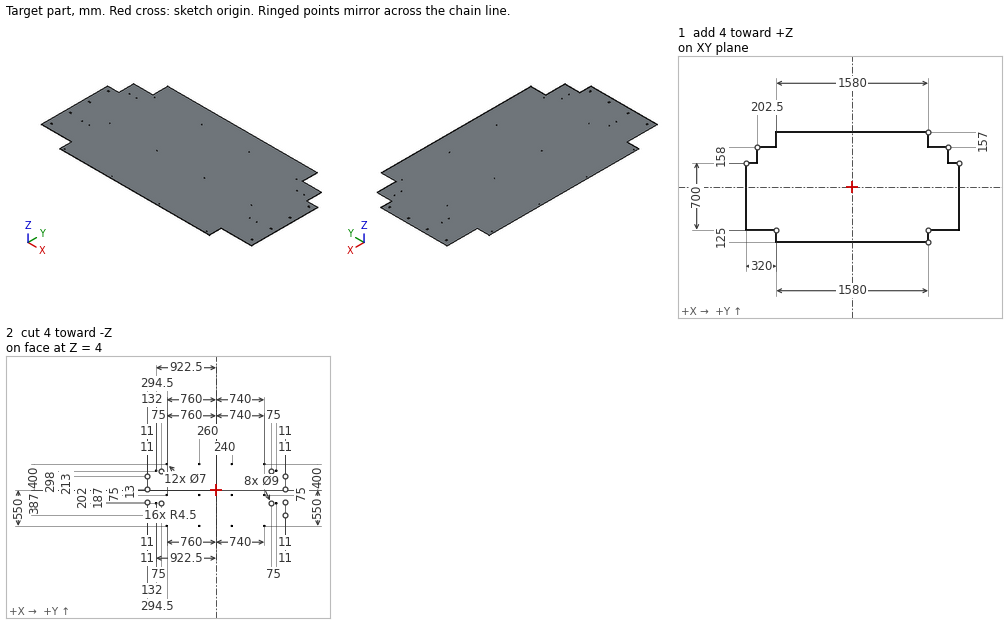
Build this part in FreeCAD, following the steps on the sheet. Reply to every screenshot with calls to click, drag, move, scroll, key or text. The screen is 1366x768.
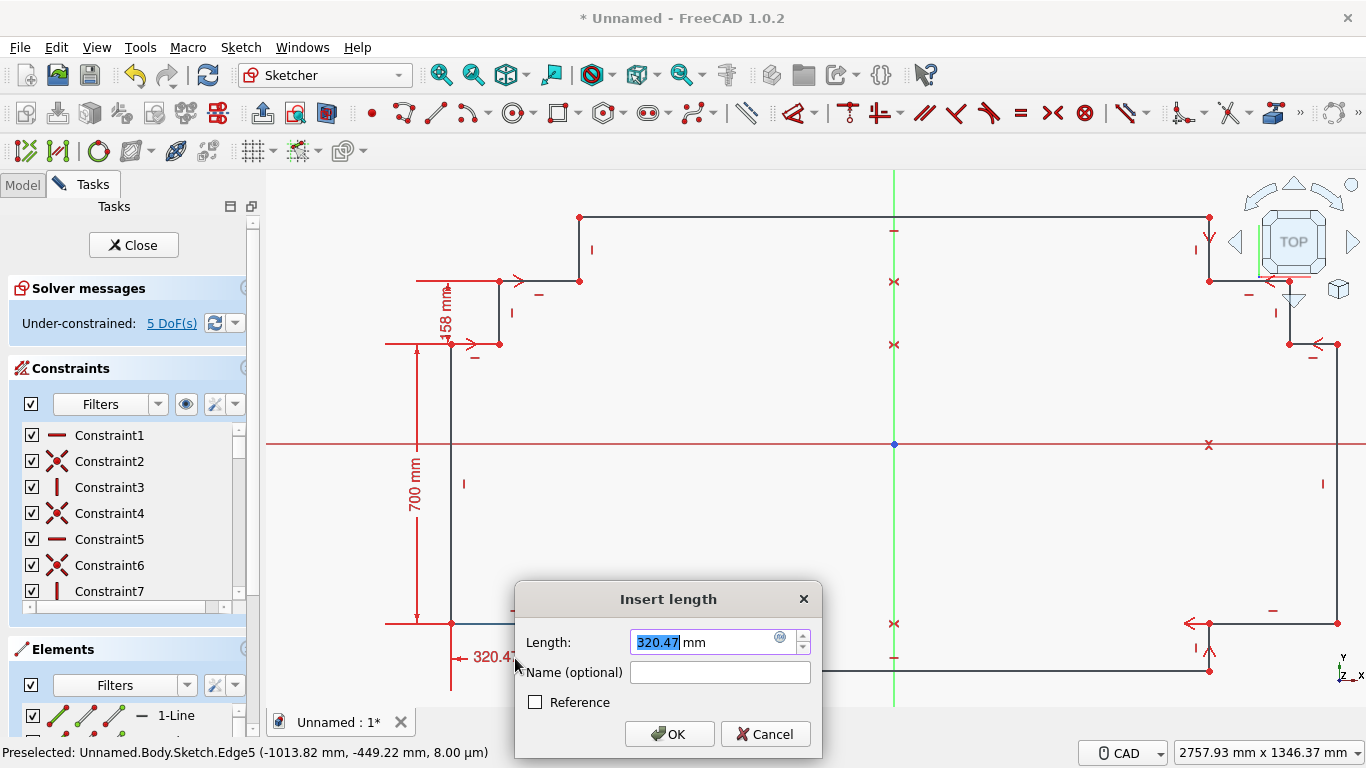
text(320)
key(Return)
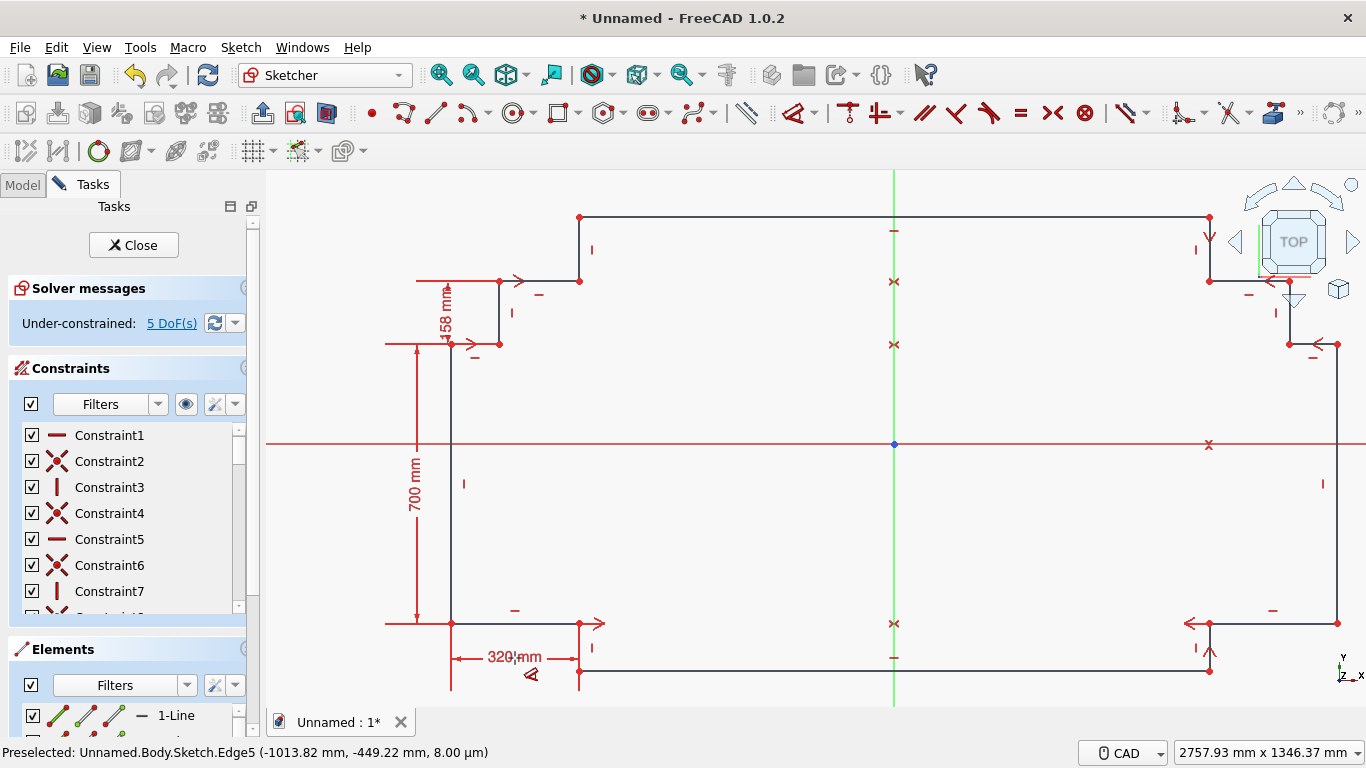
click(579, 638)
click(613, 647)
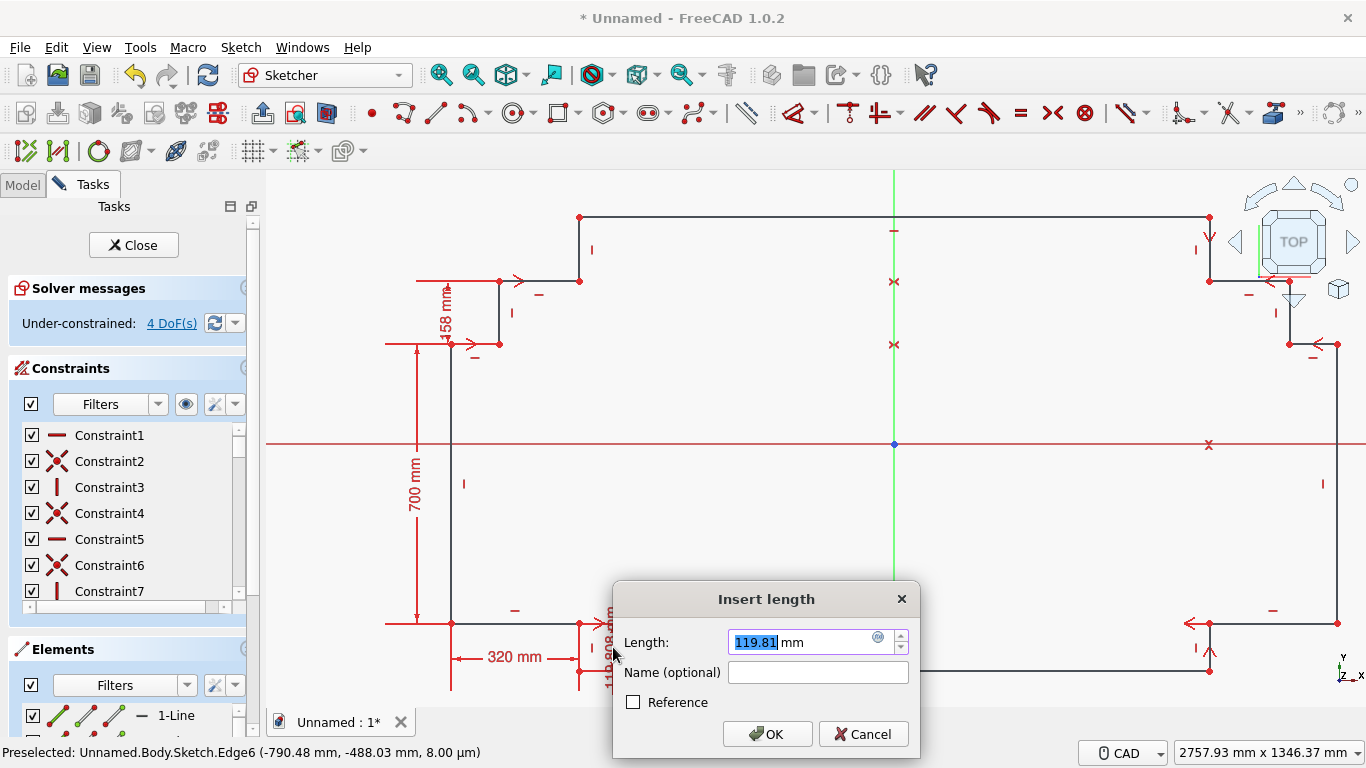
text(125)
key(Return)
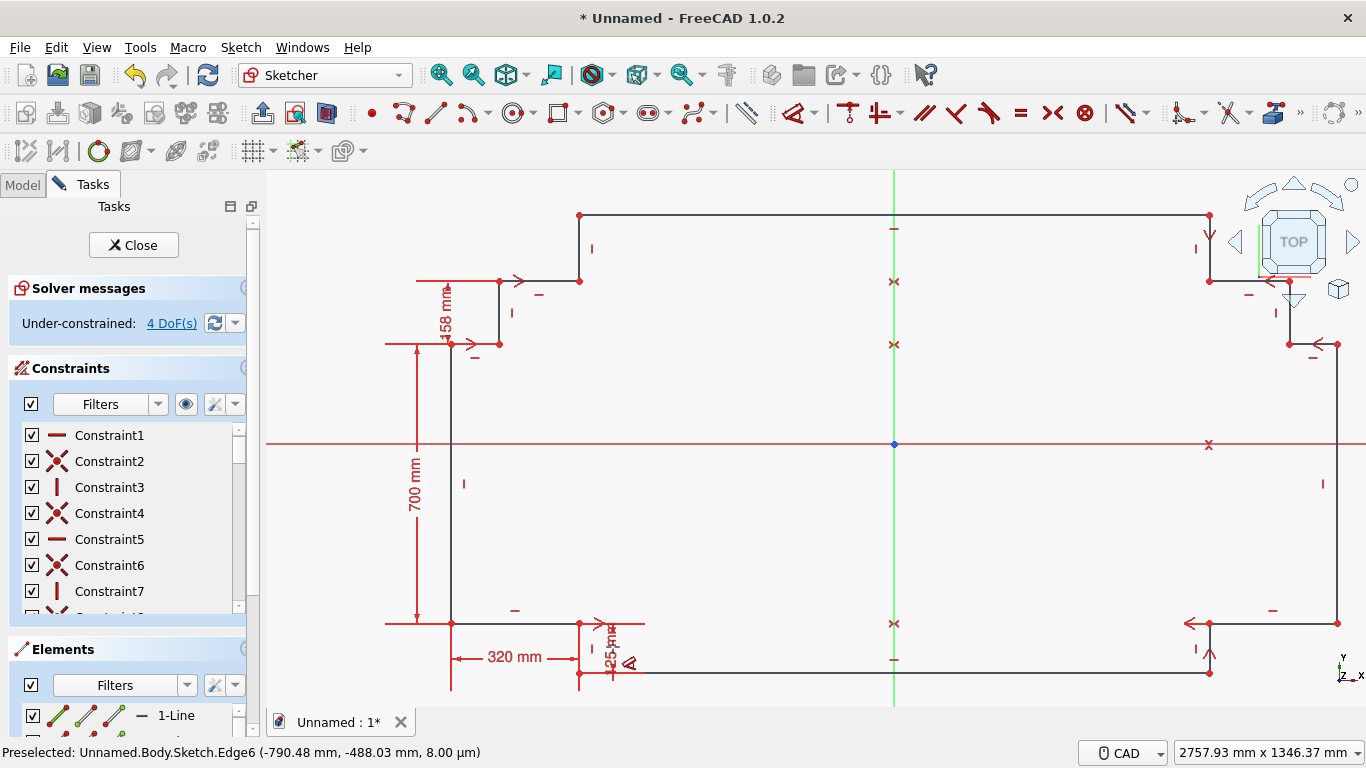
scroll(449, 427, down, 2)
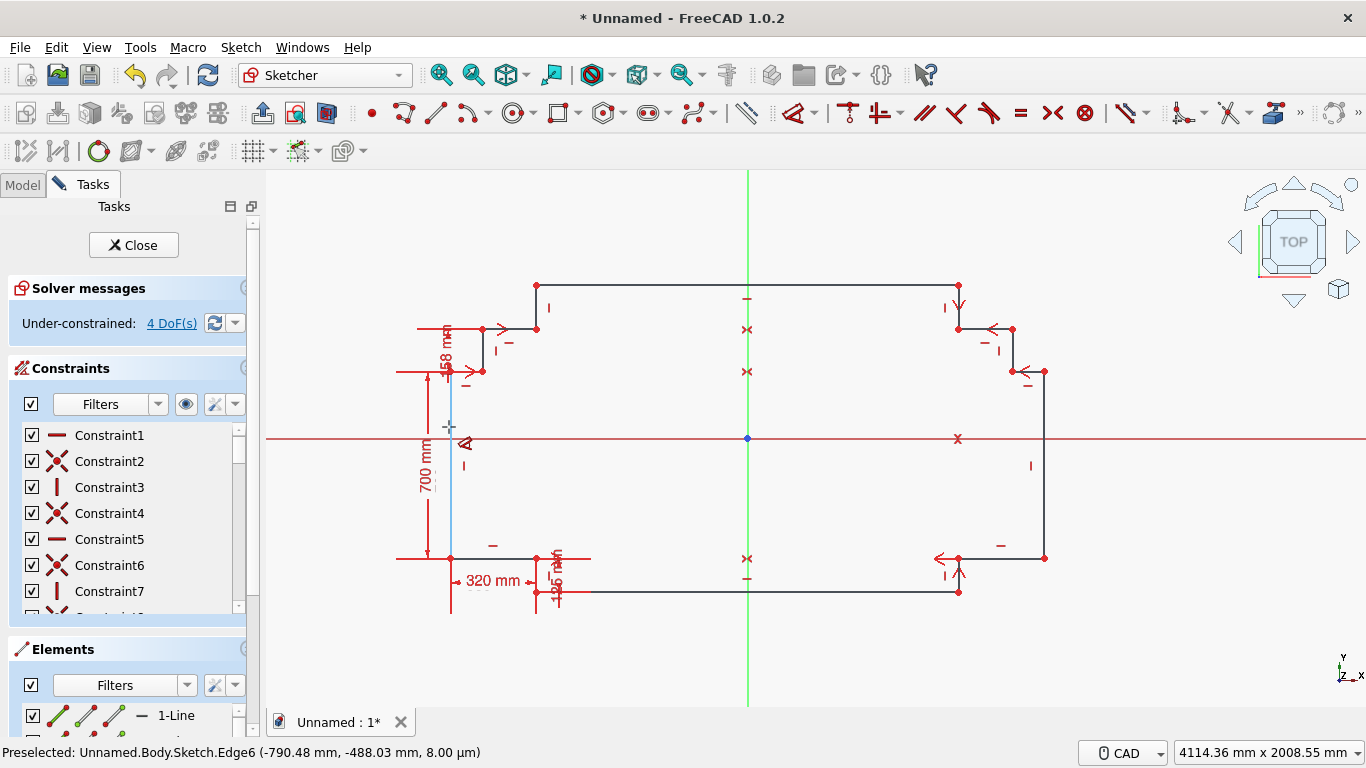
click(959, 316)
click(993, 307)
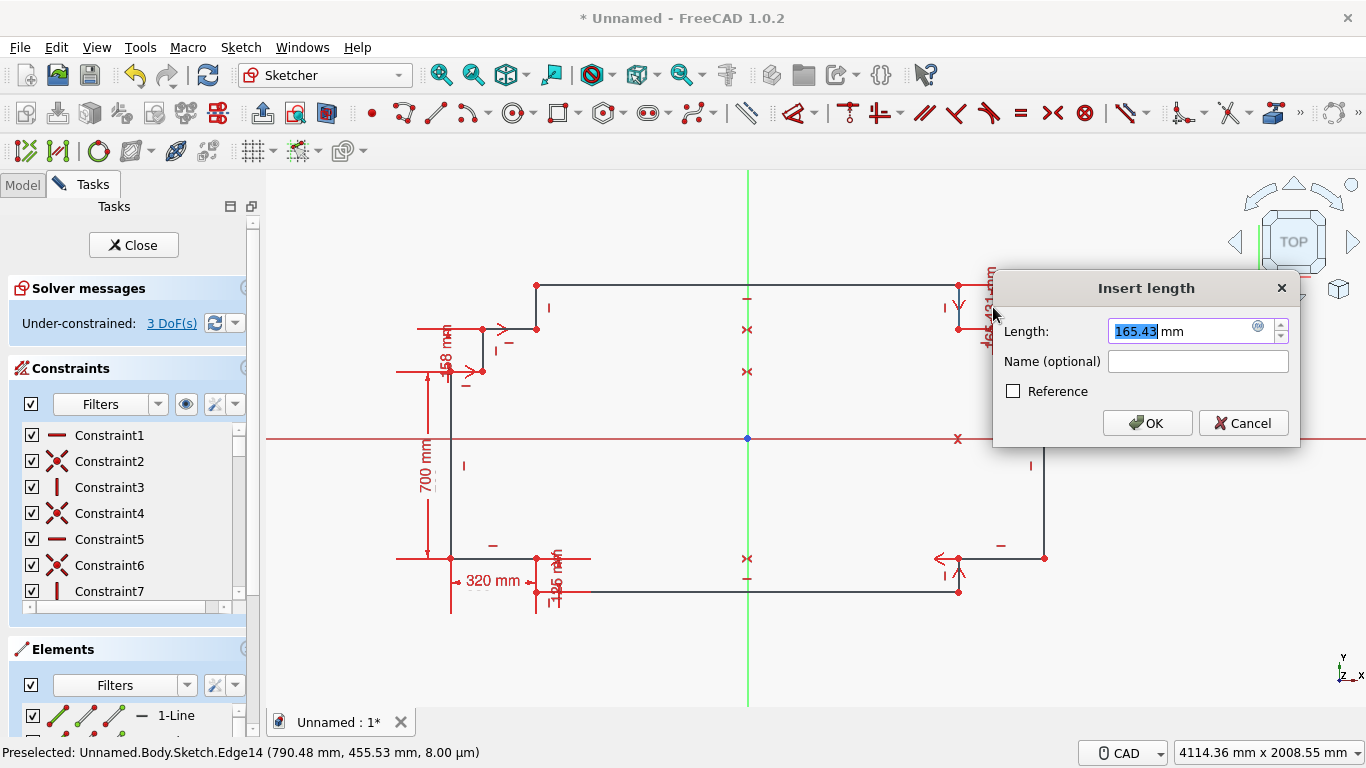
text(157)
key(Return)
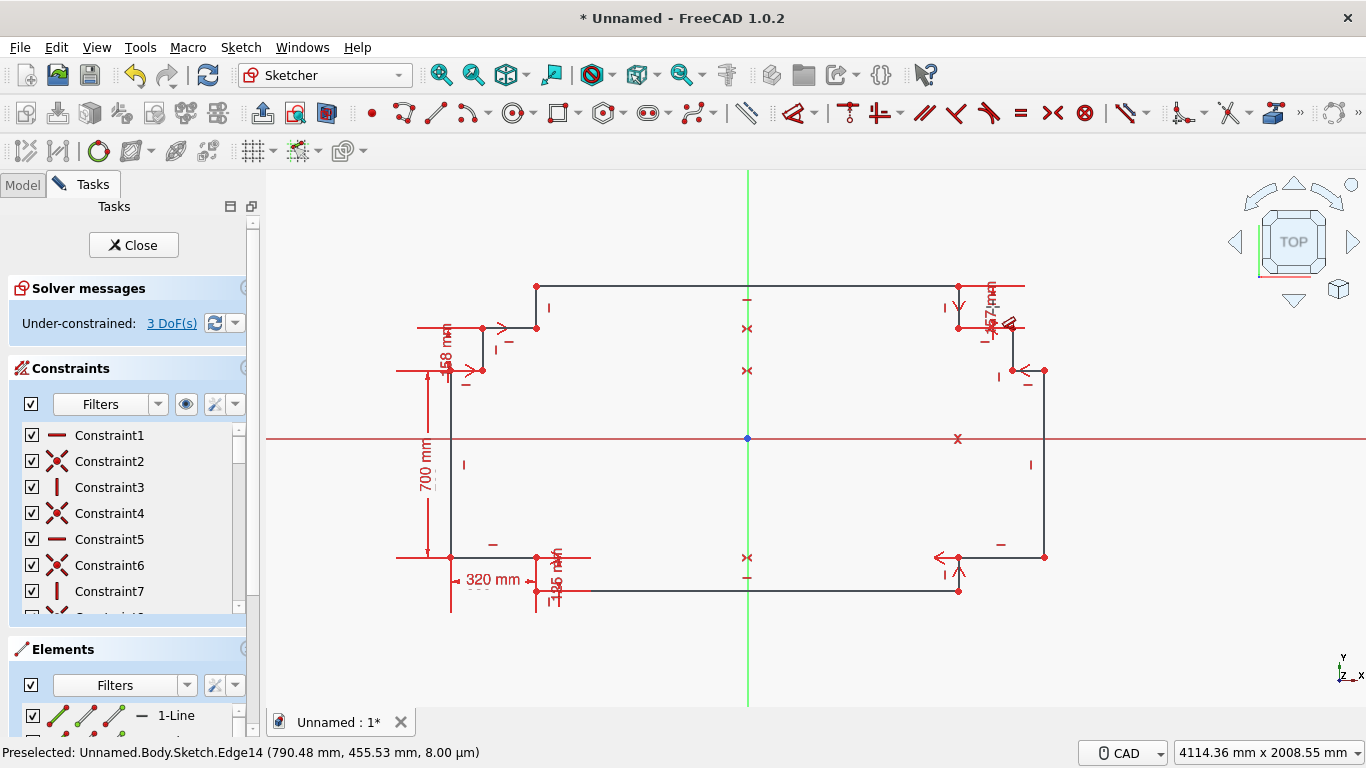
click(663, 591)
click(650, 625)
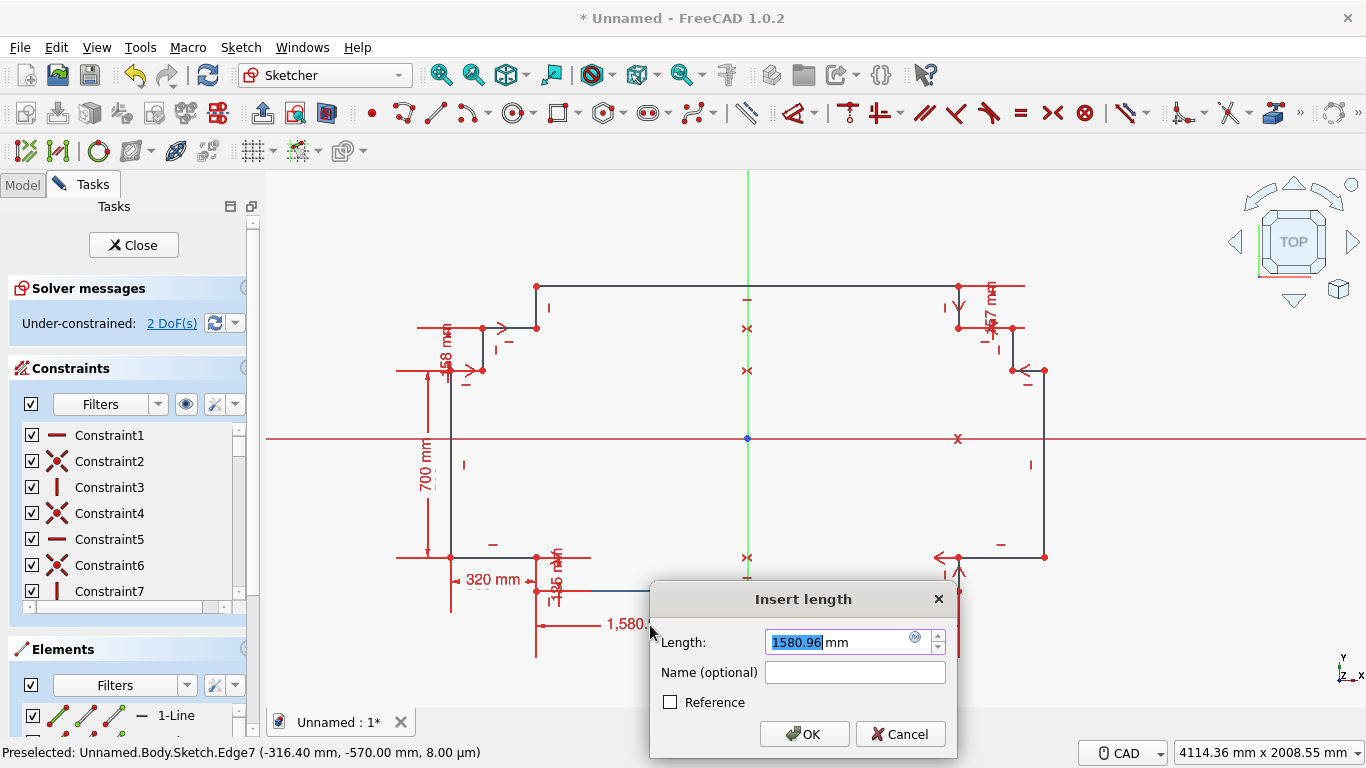
text(1580)
key(Return)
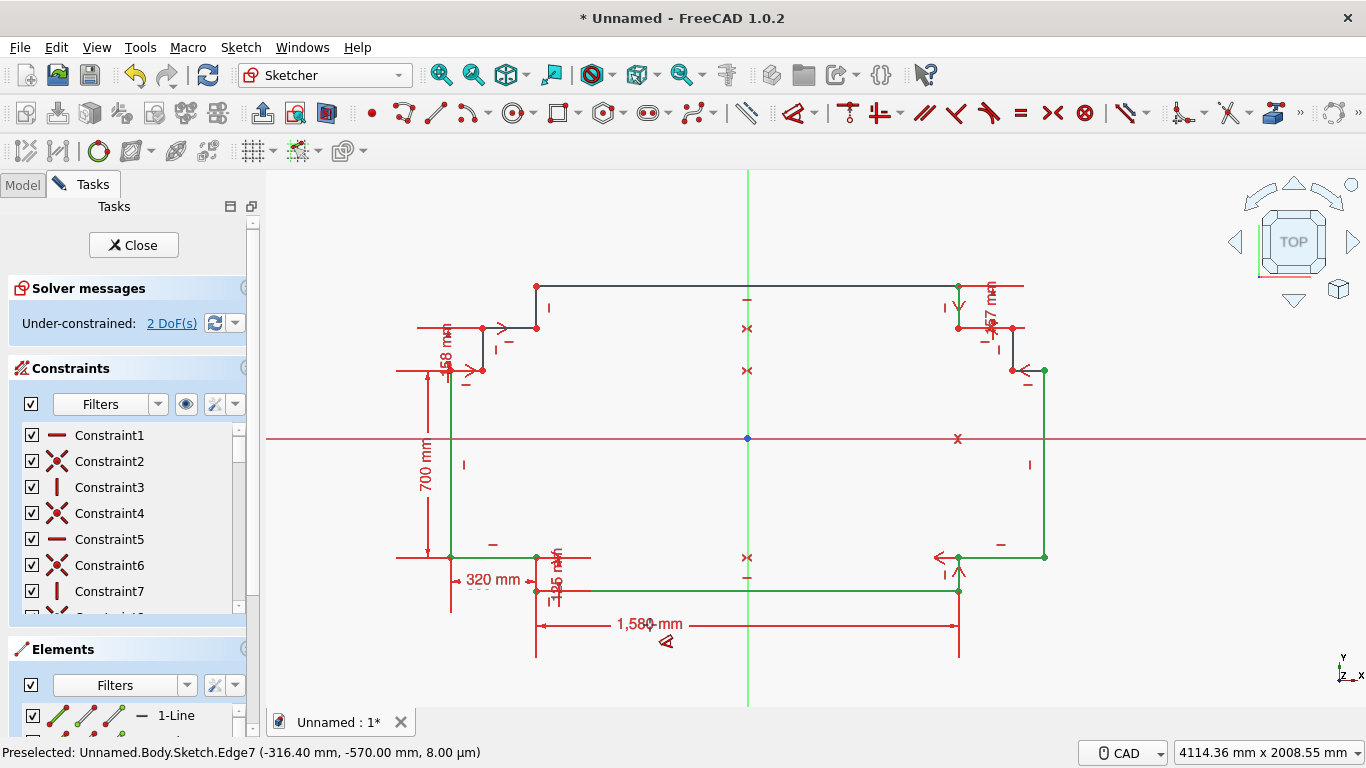
click(832, 286)
click(650, 252)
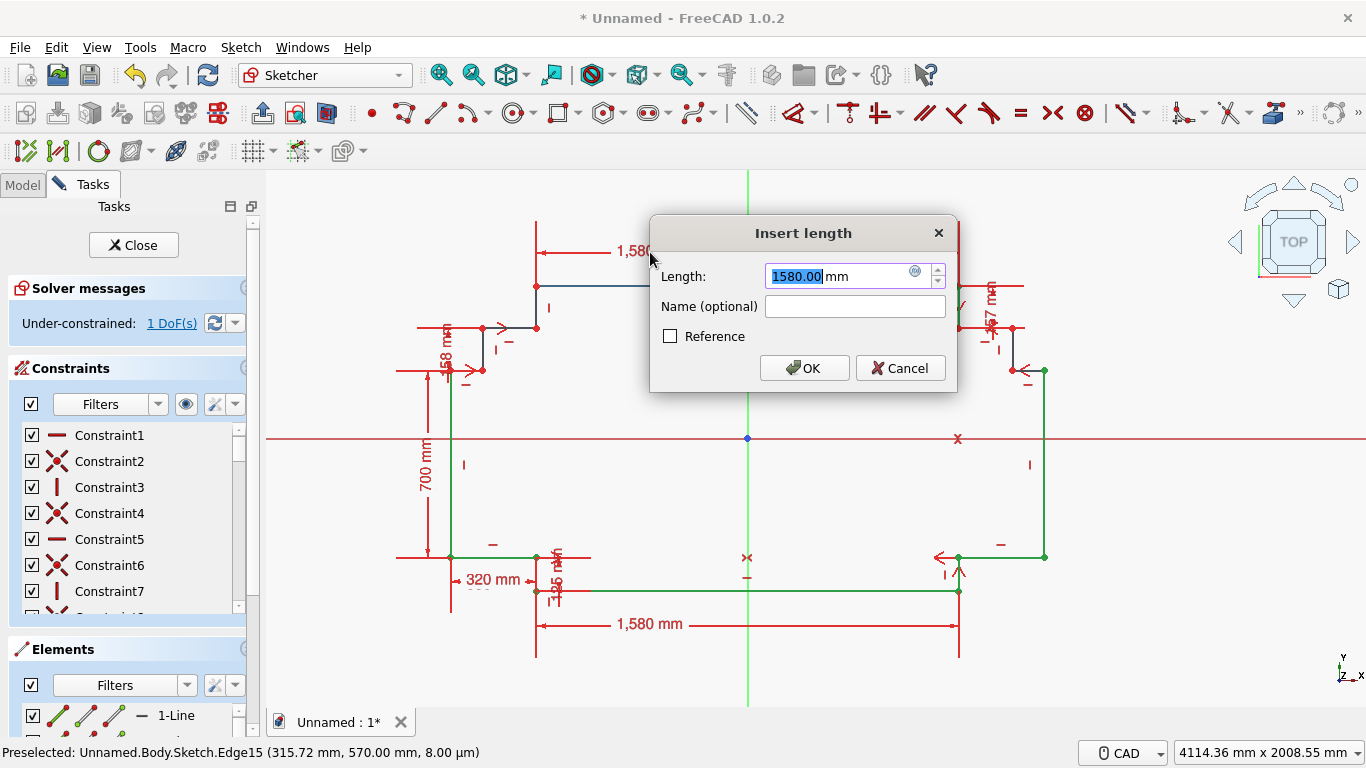
text(1580)
key(Return)